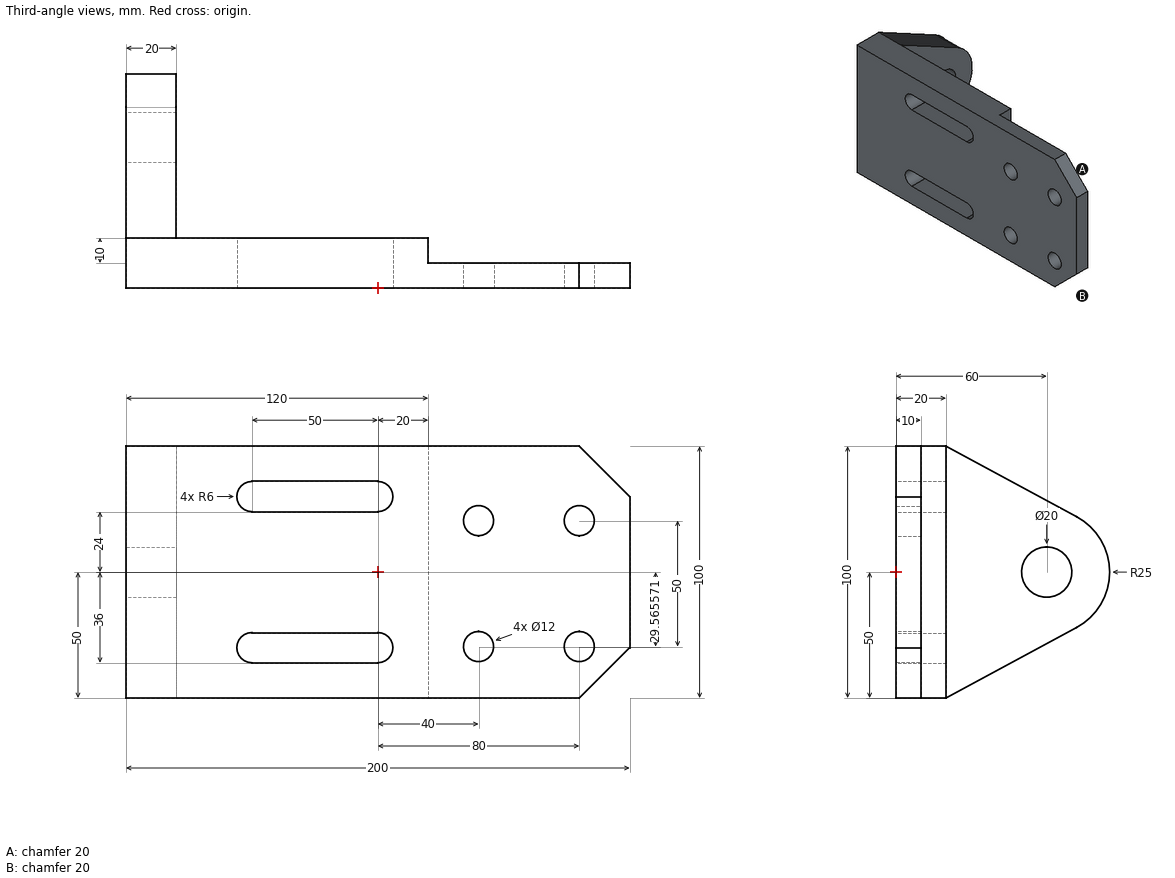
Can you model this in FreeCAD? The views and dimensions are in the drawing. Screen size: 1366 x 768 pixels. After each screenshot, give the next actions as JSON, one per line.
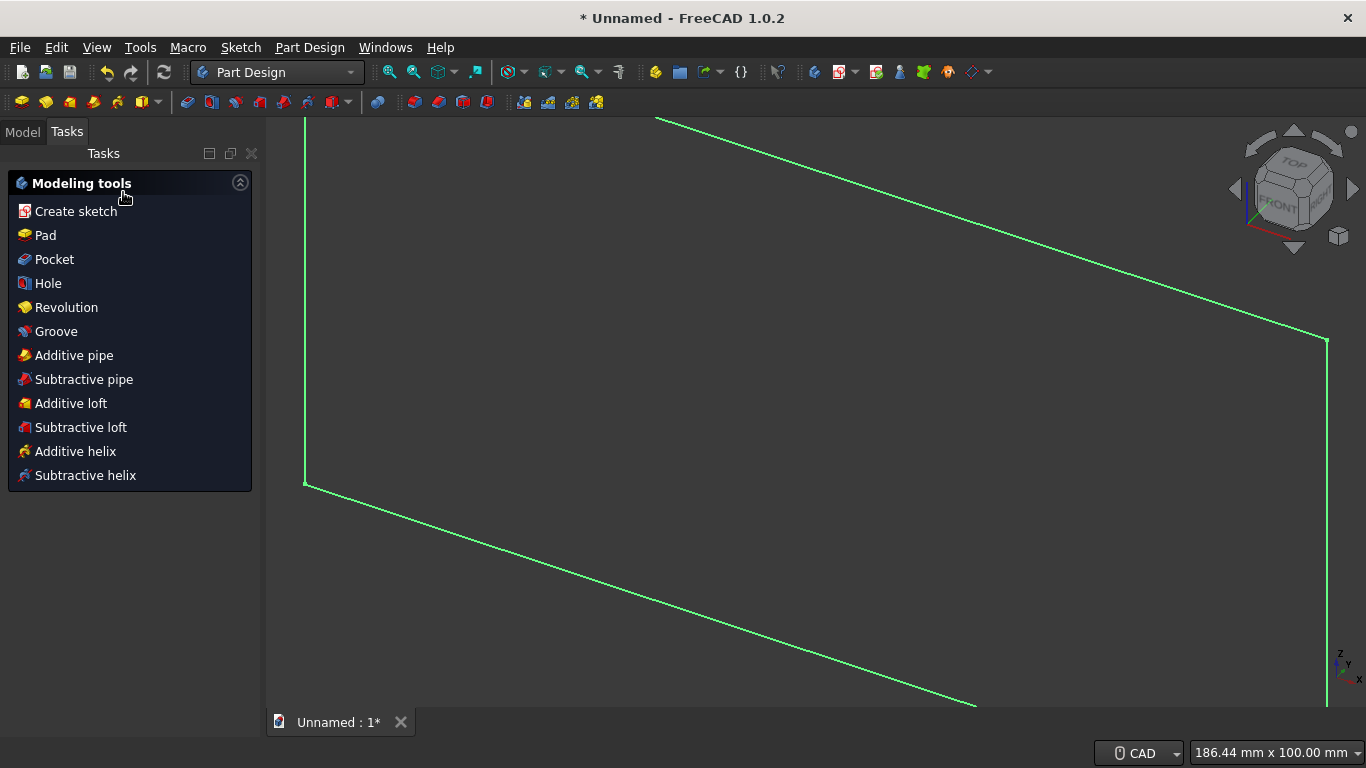
{"action": "left_click", "coordinate": [22, 102]}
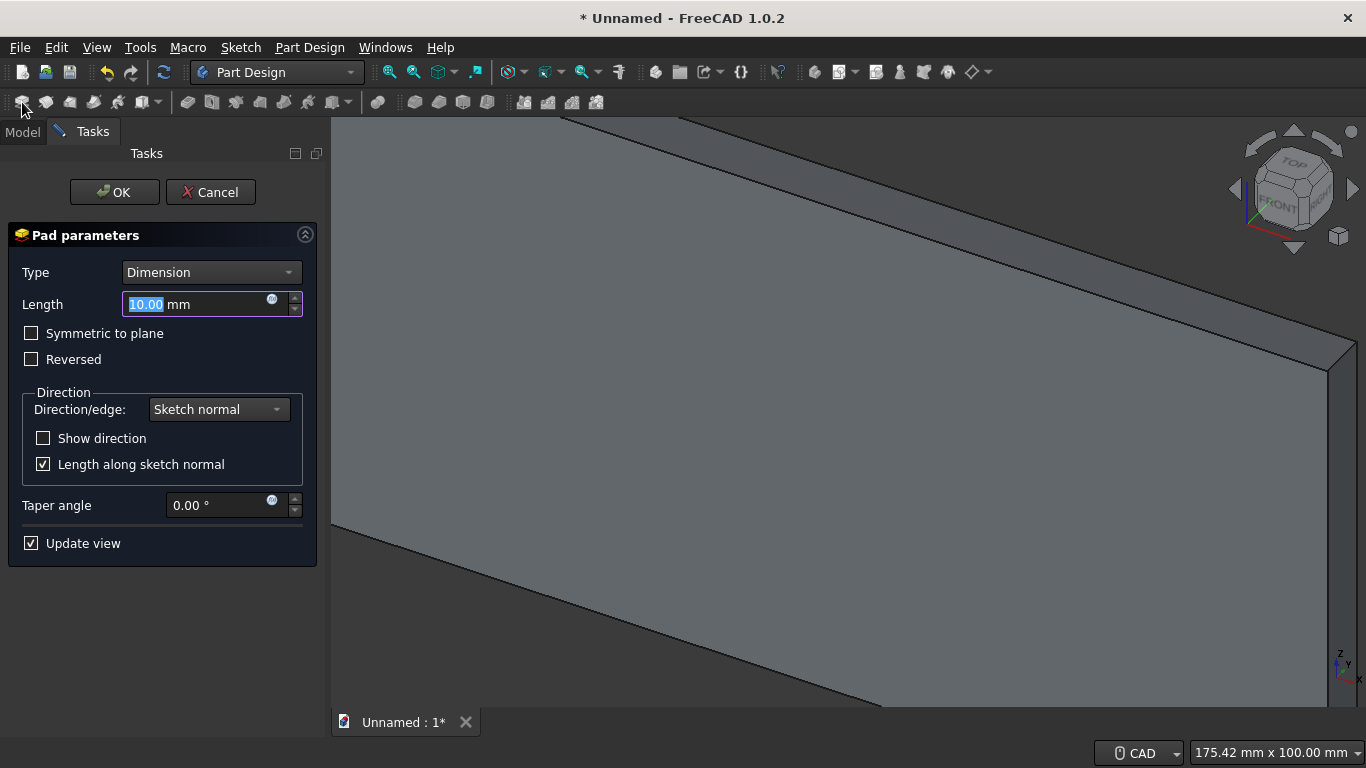
{"action": "type", "text": "10"}
{"action": "key", "text": "Tab"}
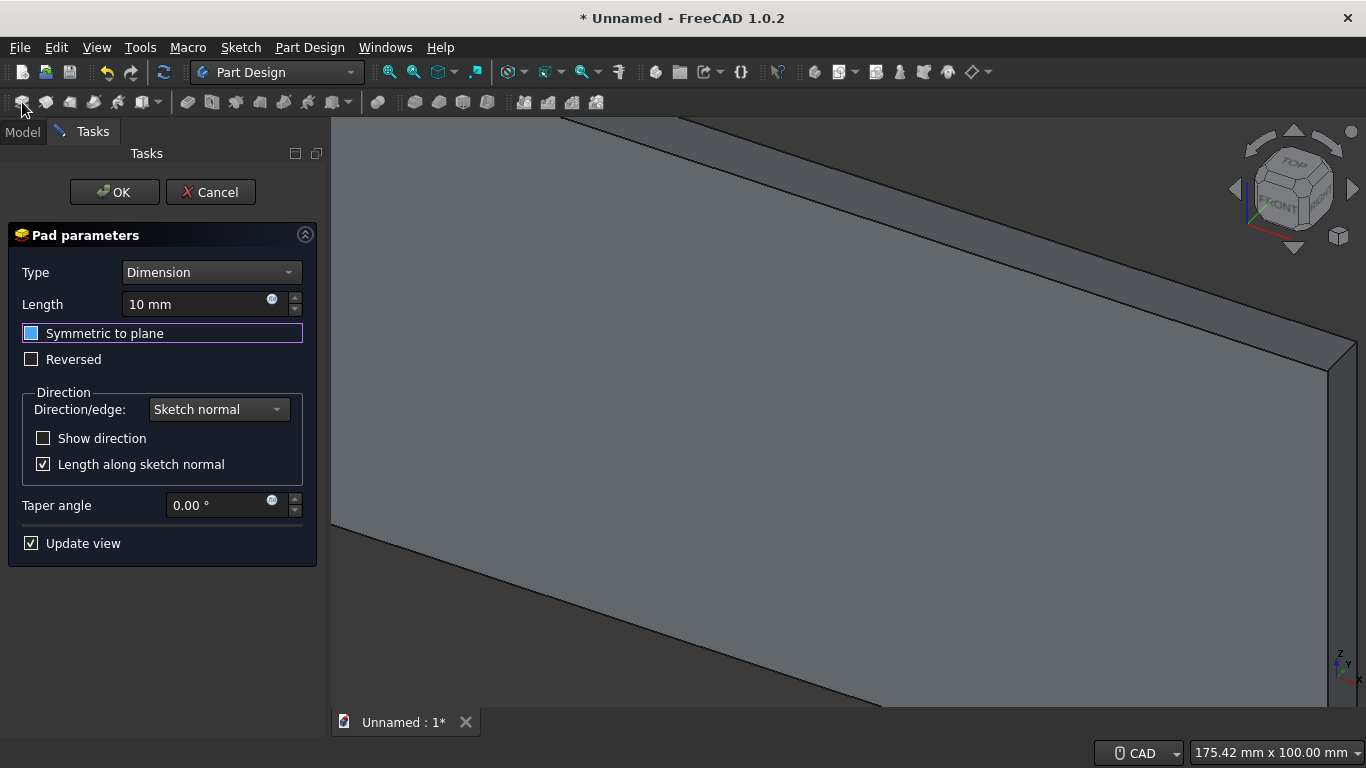
{"action": "left_click", "coordinate": [30, 359]}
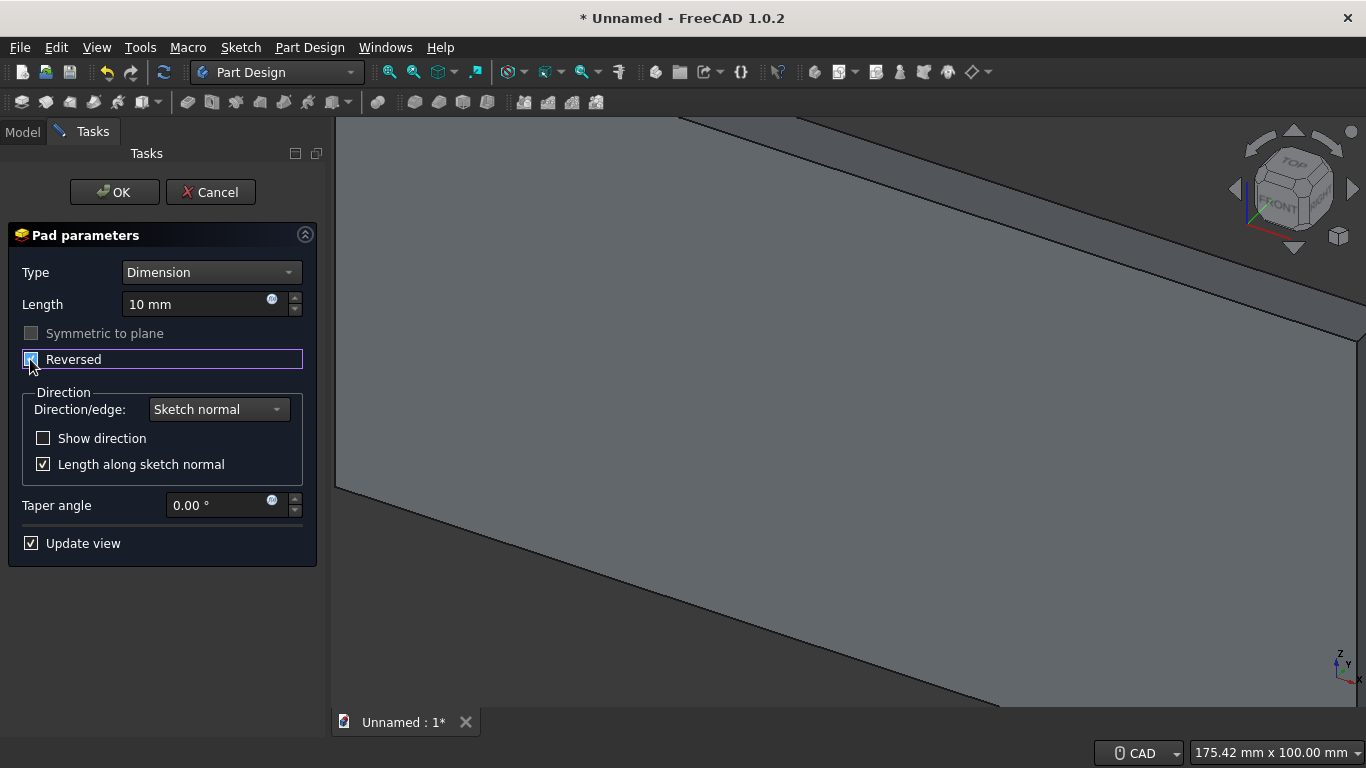
{"action": "left_click", "coordinate": [115, 192]}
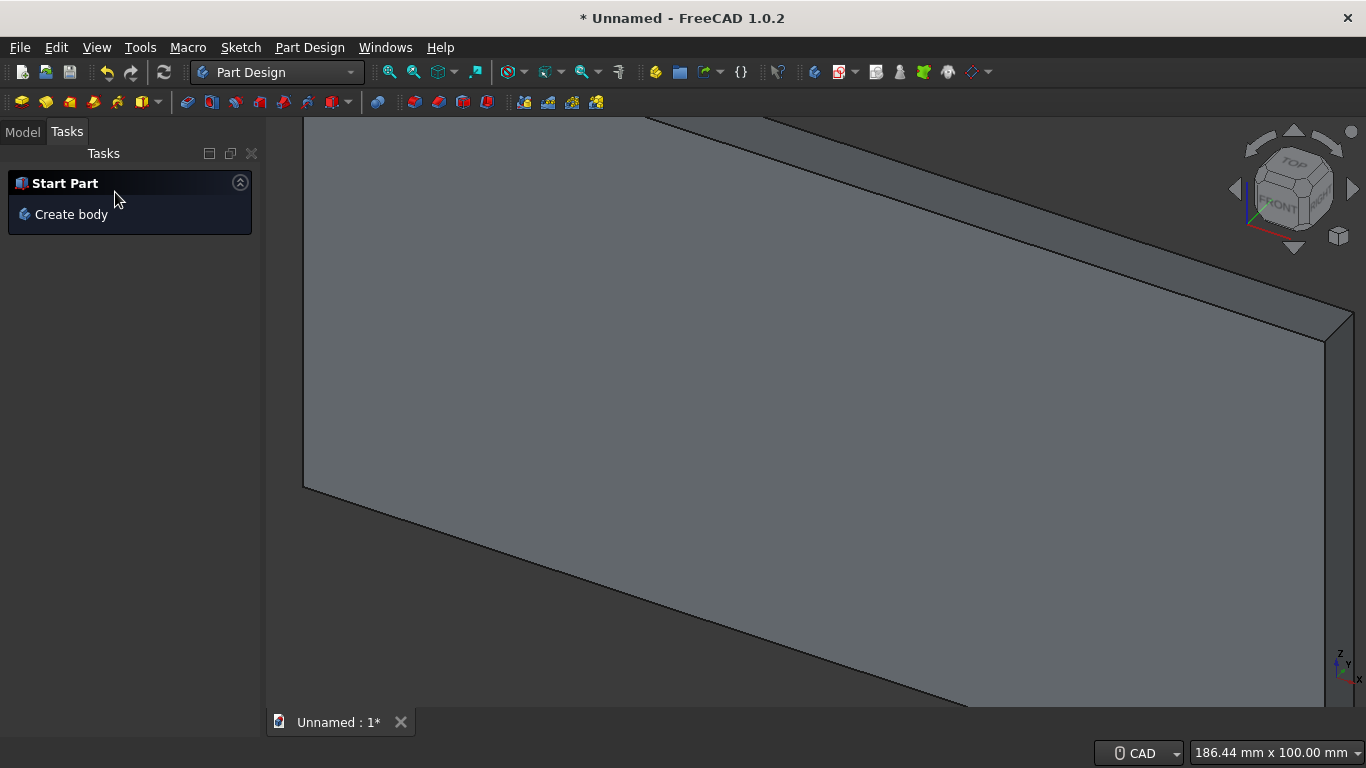
{"action": "left_click", "coordinate": [390, 72]}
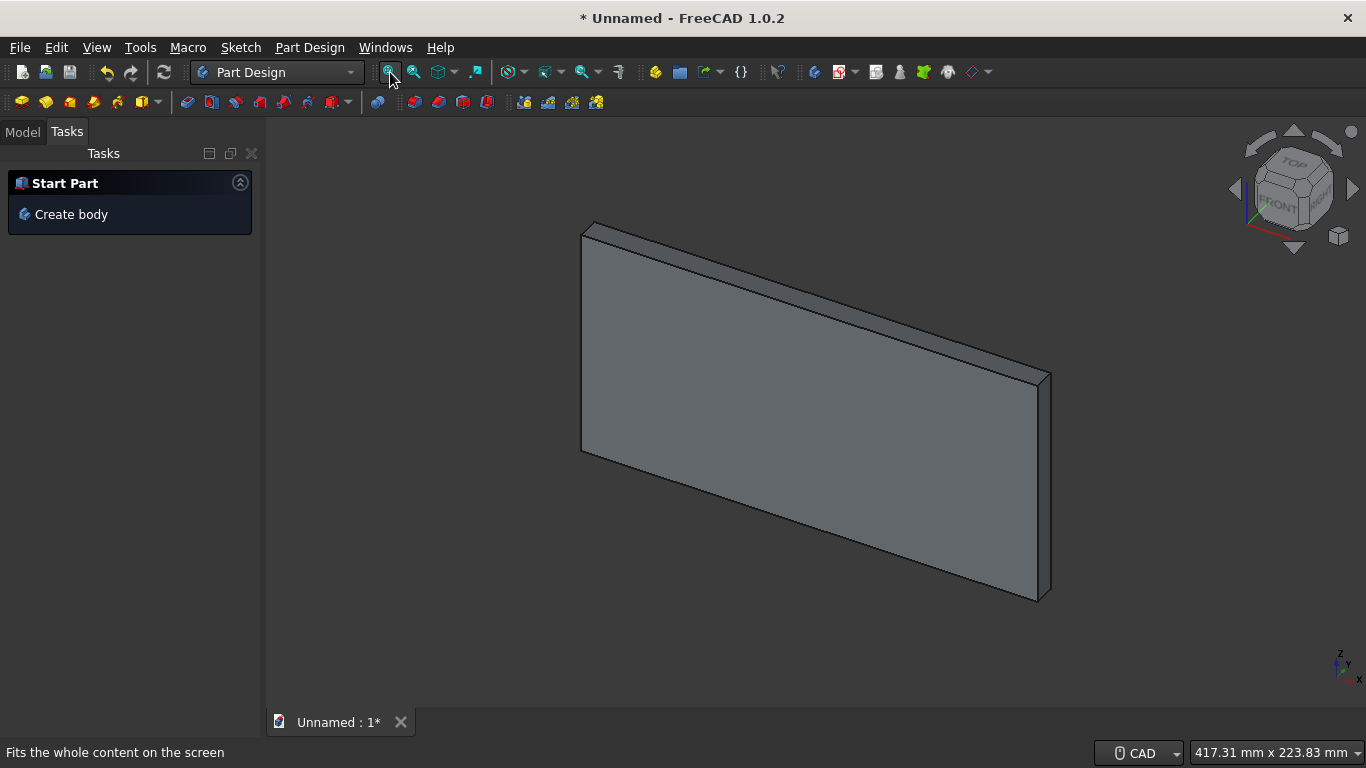
{"action": "key", "text": "4"}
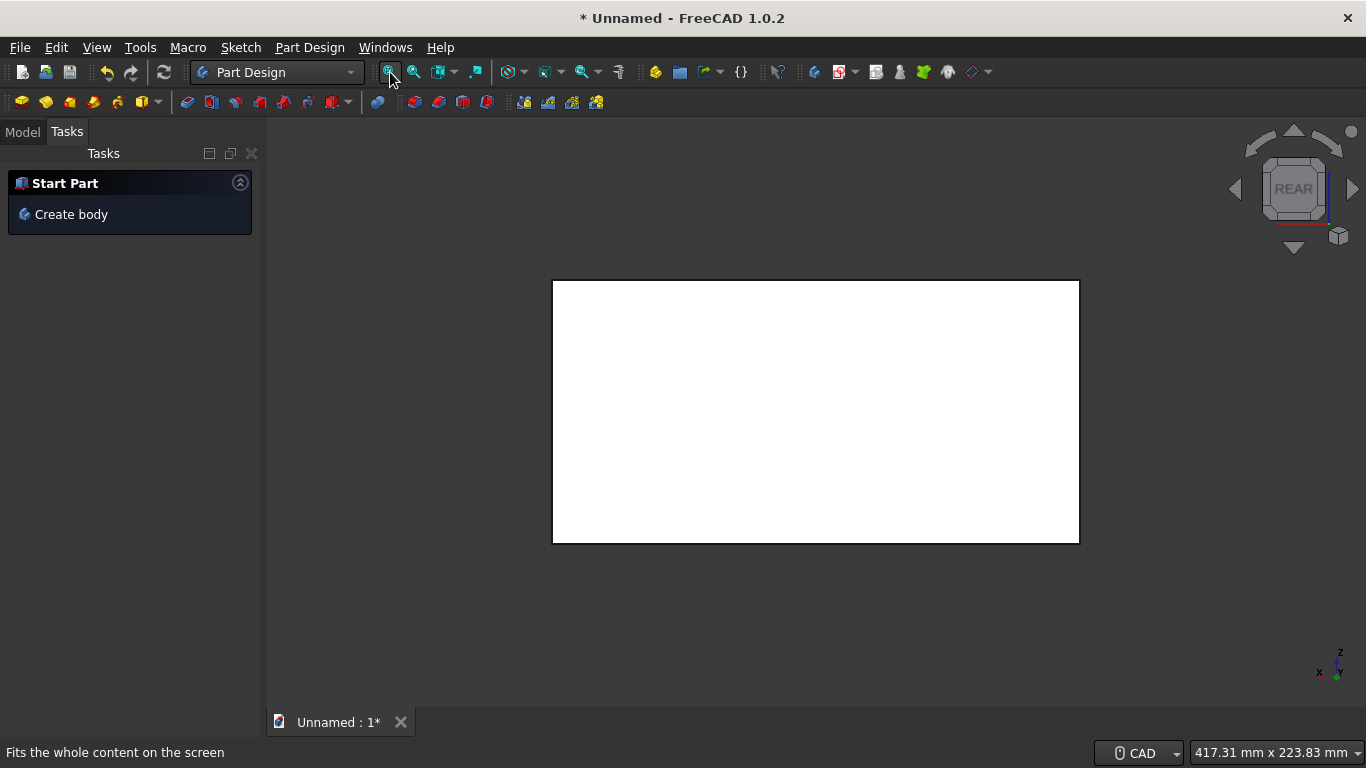
{"action": "left_click", "coordinate": [741, 411]}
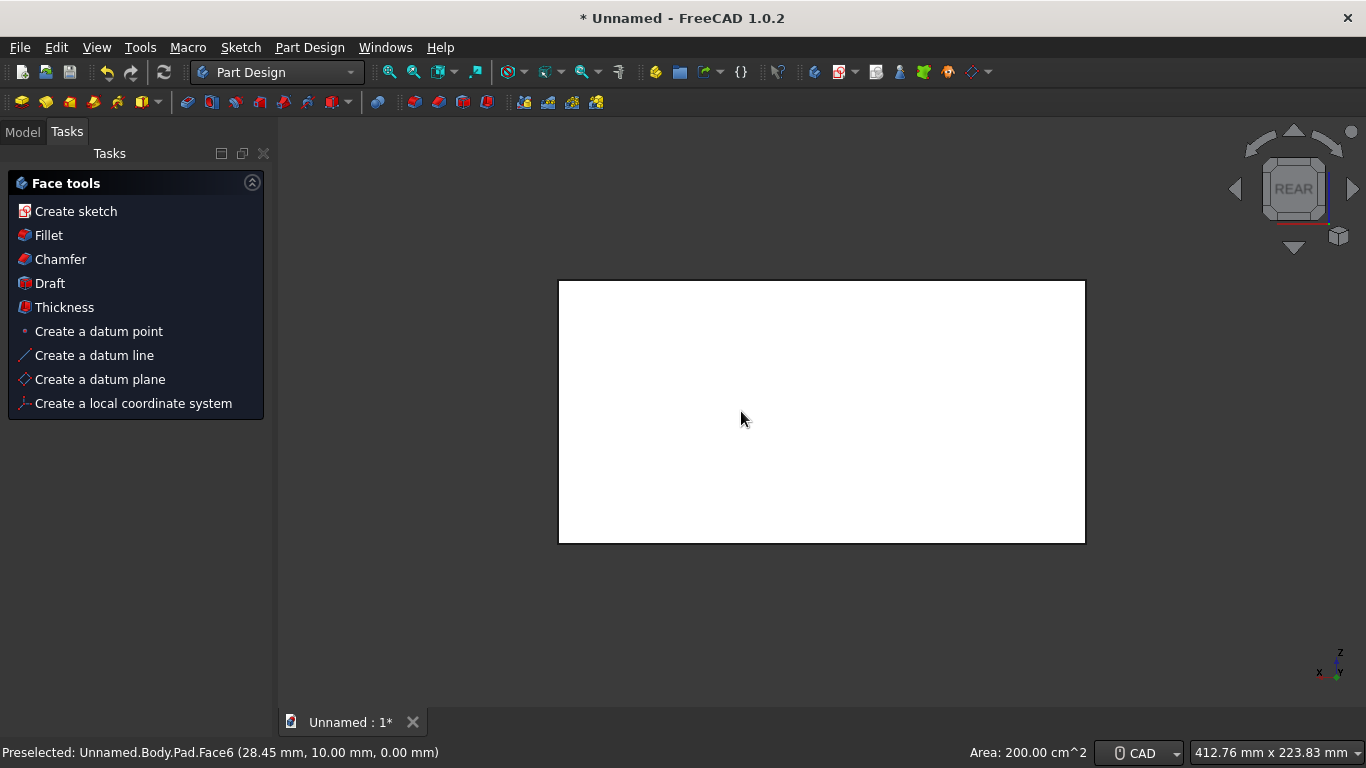
{"action": "left_click", "coordinate": [840, 72]}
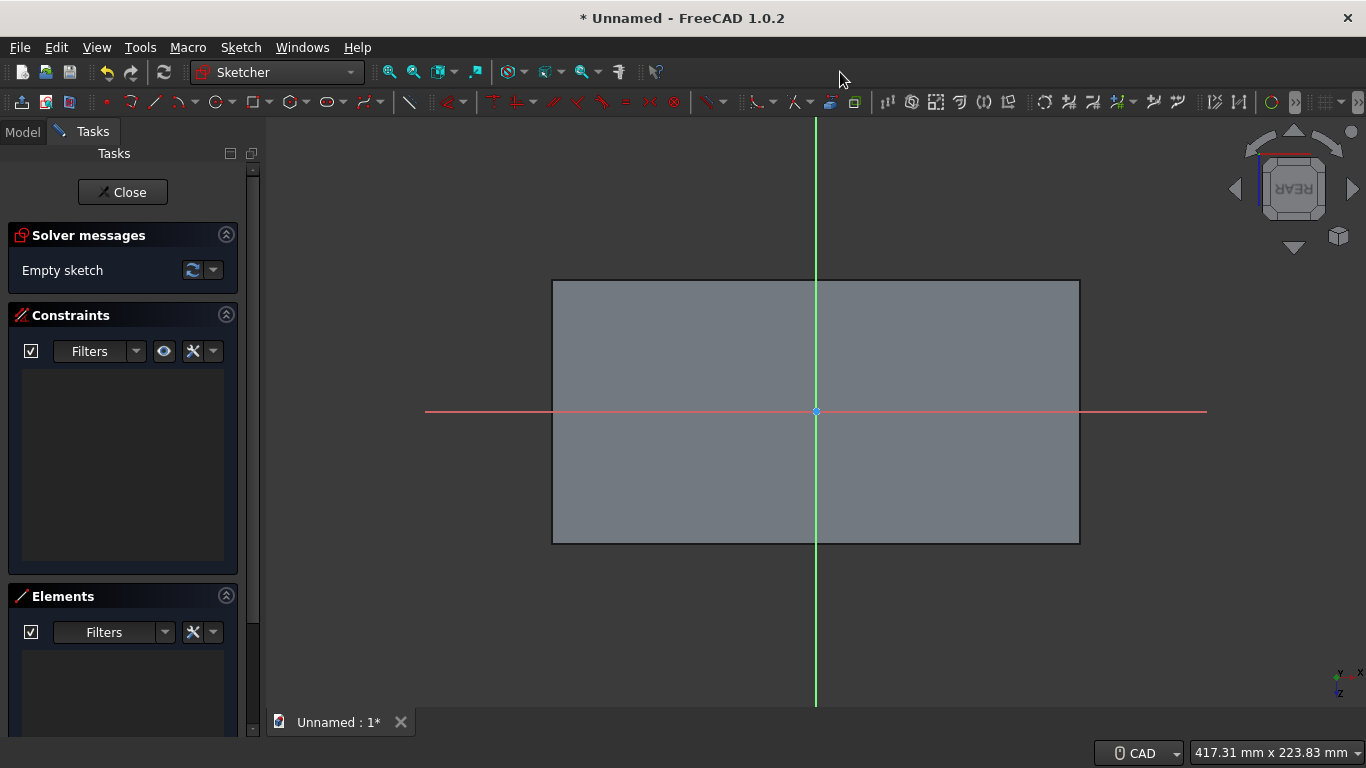
{"action": "scroll", "coordinate": [635, 412], "scroll_direction": "up", "scroll_amount": 2}